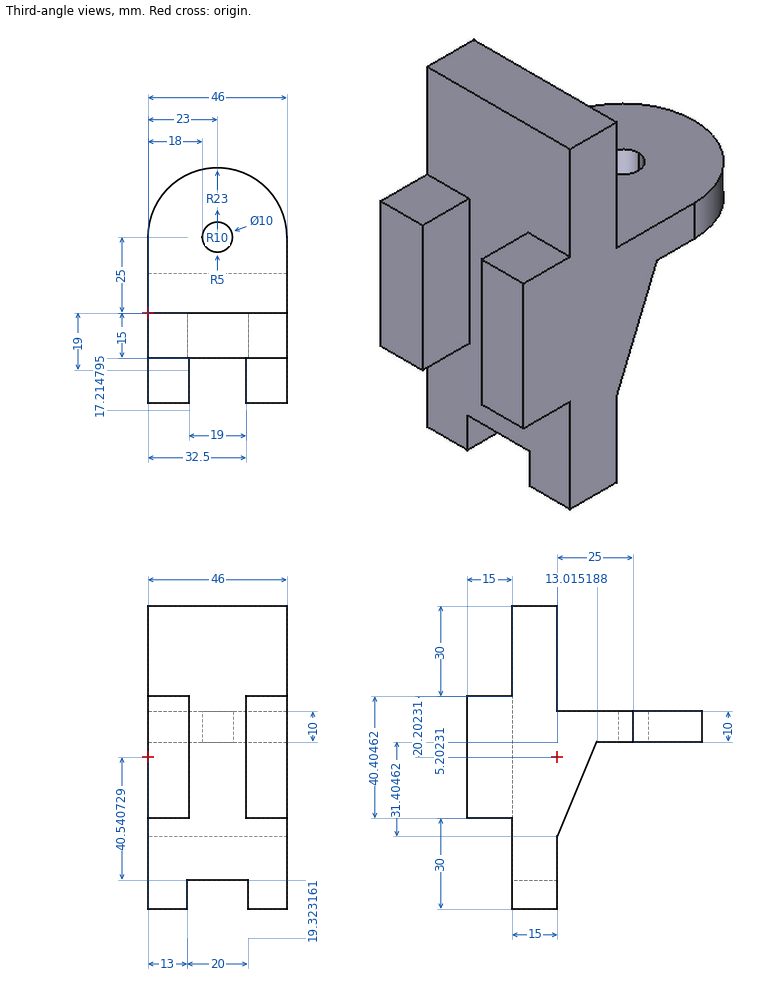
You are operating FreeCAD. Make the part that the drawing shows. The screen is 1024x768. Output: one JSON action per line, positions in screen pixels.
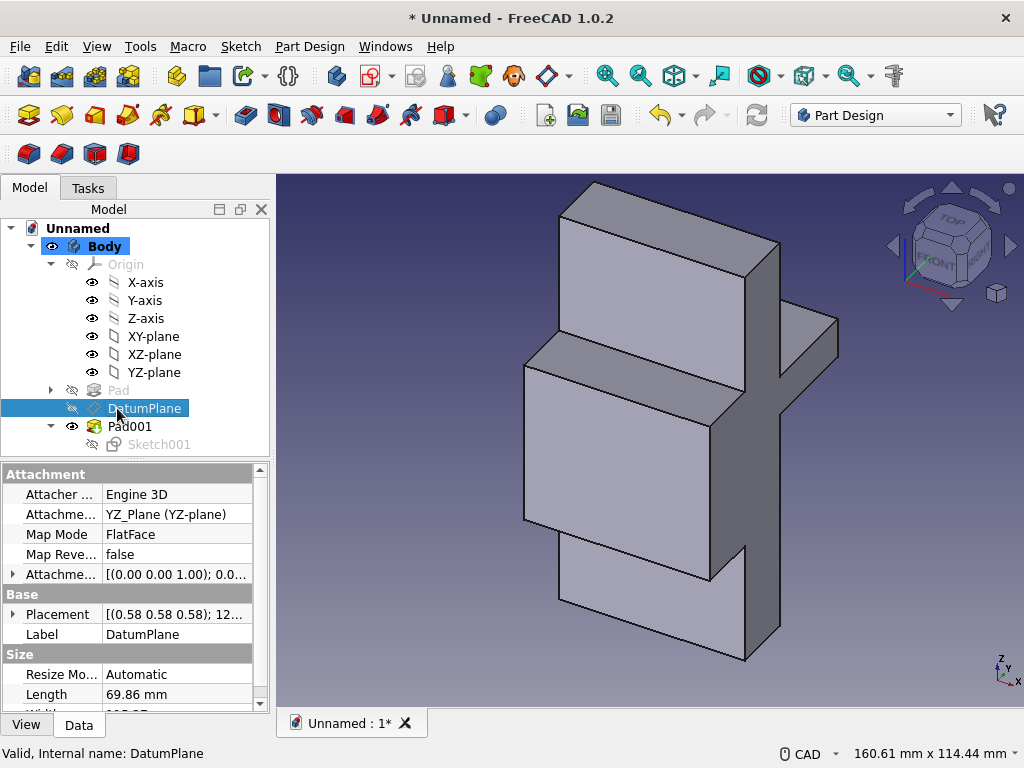
{"action": "left_click", "coordinate": [608, 76]}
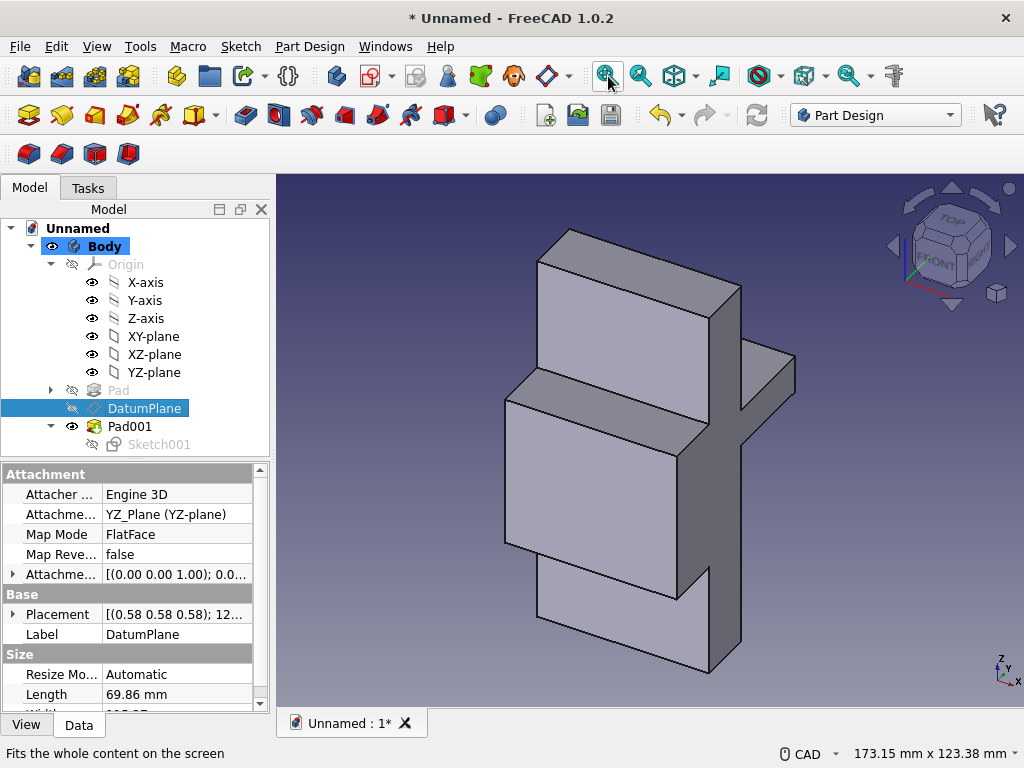
{"action": "left_click", "coordinate": [137, 372]}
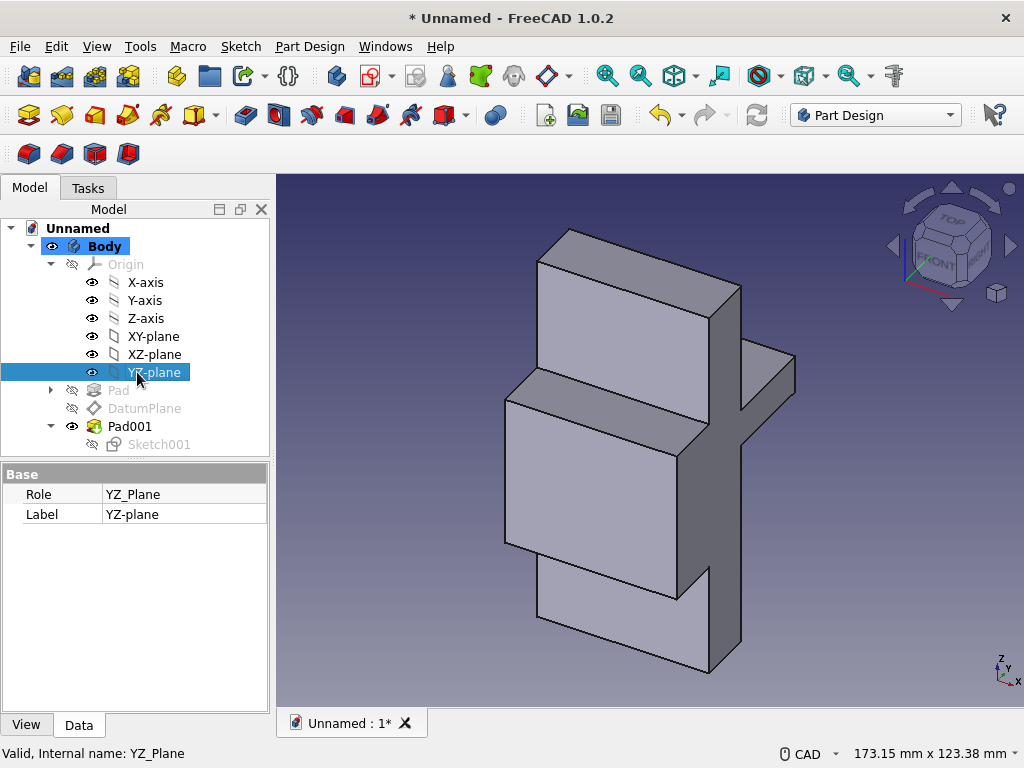
{"action": "left_click", "coordinate": [546, 76]}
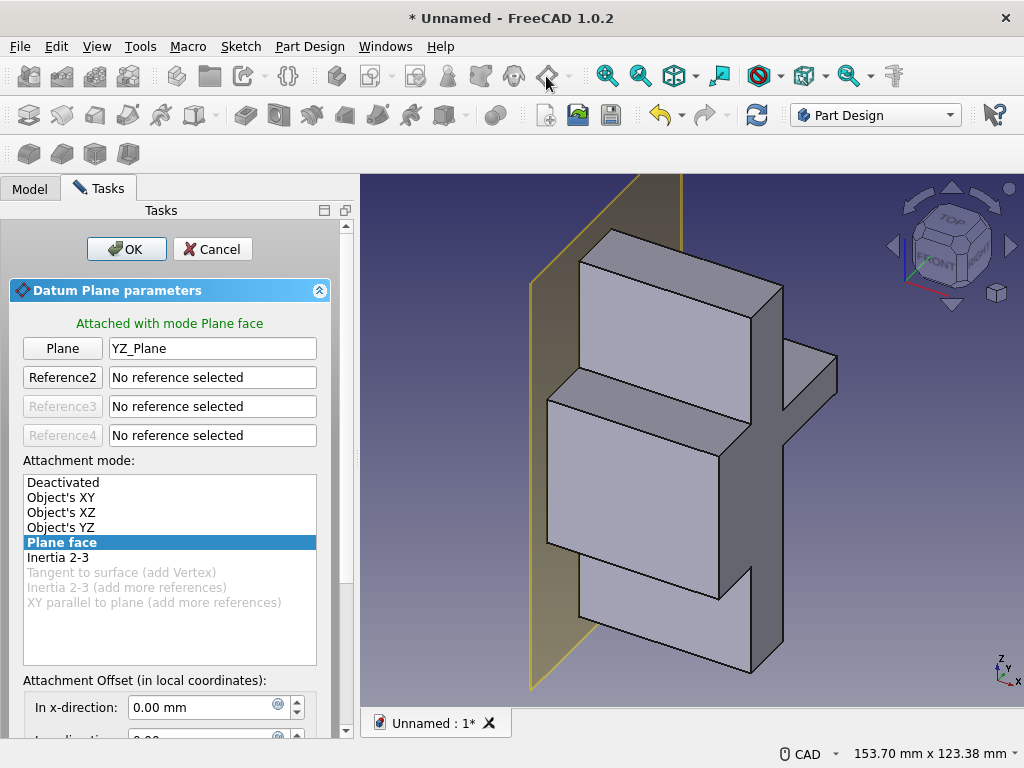
{"action": "scroll", "coordinate": [346, 479], "scroll_direction": "down", "scroll_amount": 2}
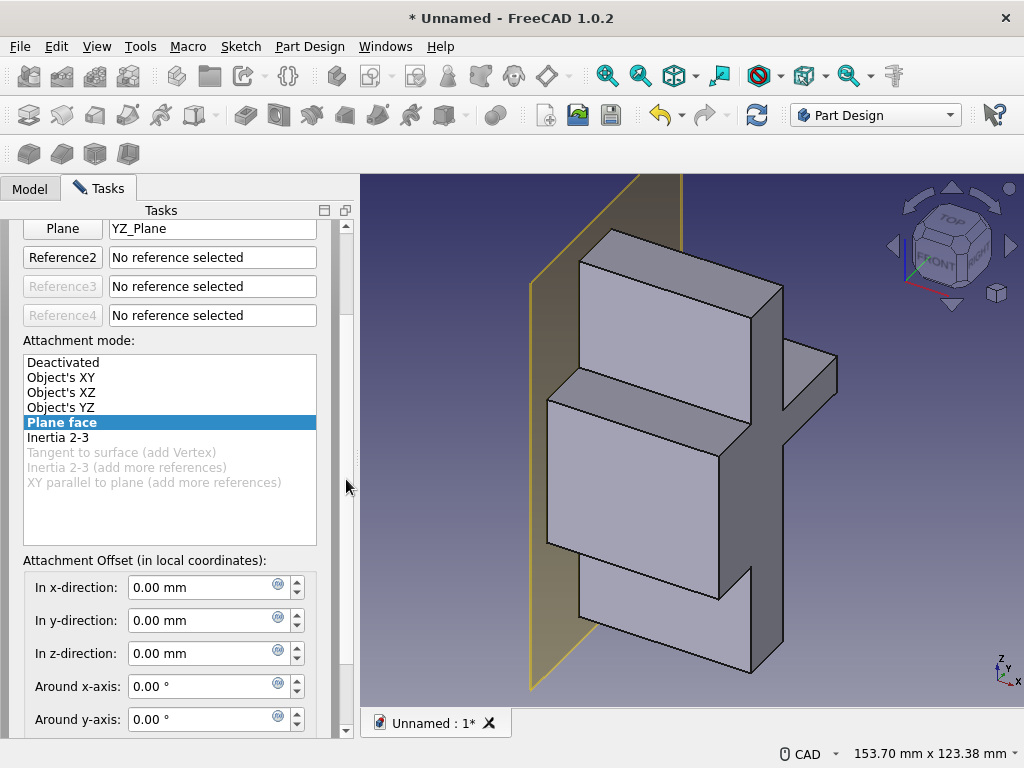
{"action": "triple_click", "coordinate": [210, 654]}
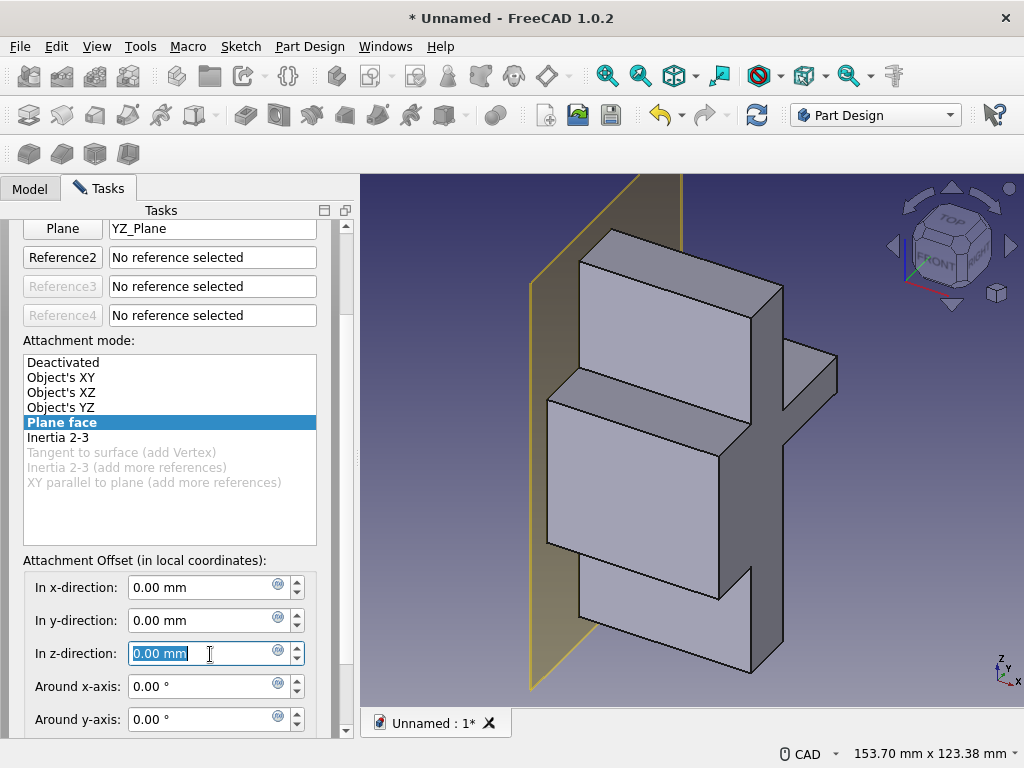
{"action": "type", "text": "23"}
{"action": "key", "text": "Tab"}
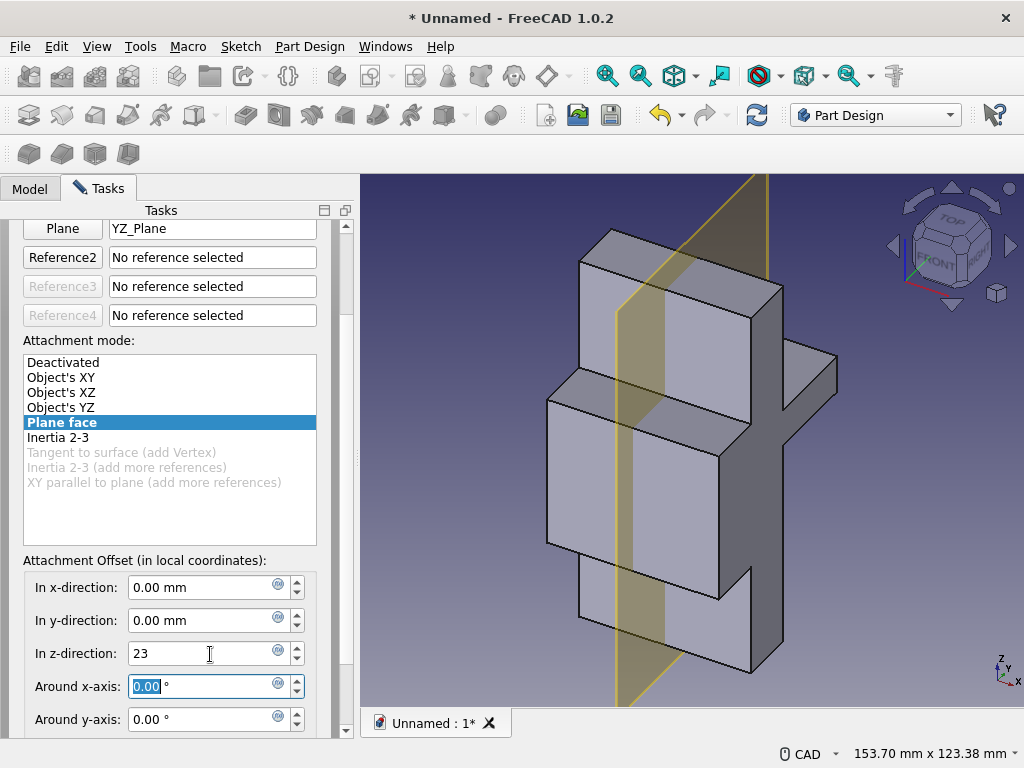
{"action": "scroll", "coordinate": [346, 479], "scroll_direction": "up", "scroll_amount": 3}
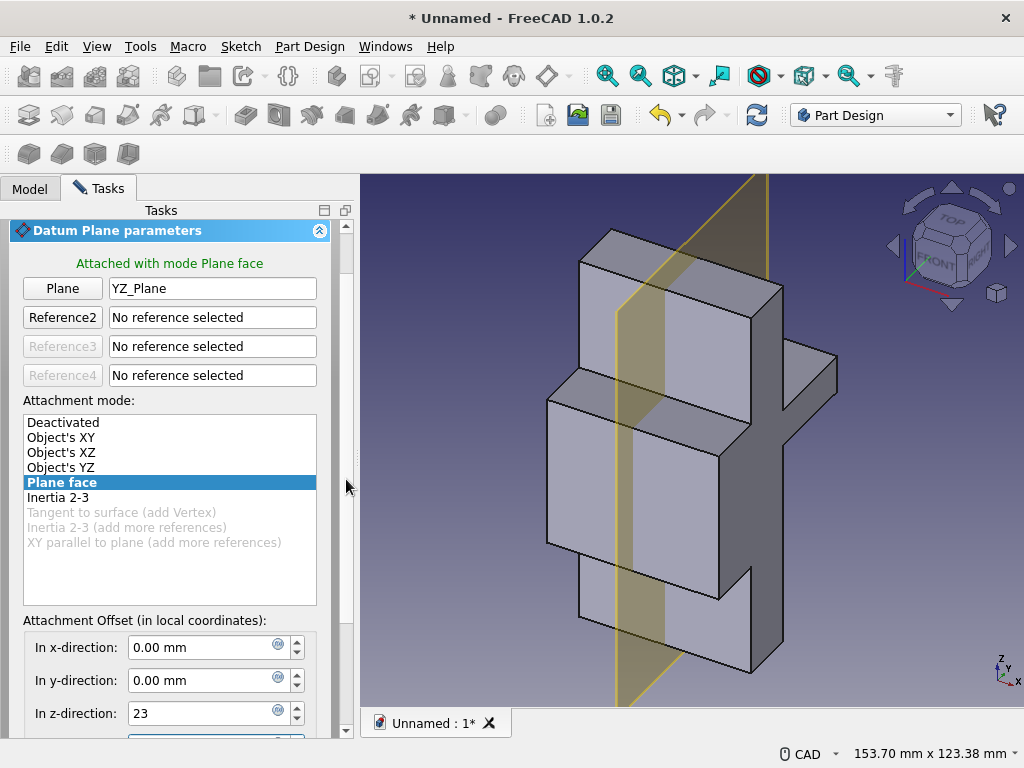
{"action": "left_click", "coordinate": [127, 249]}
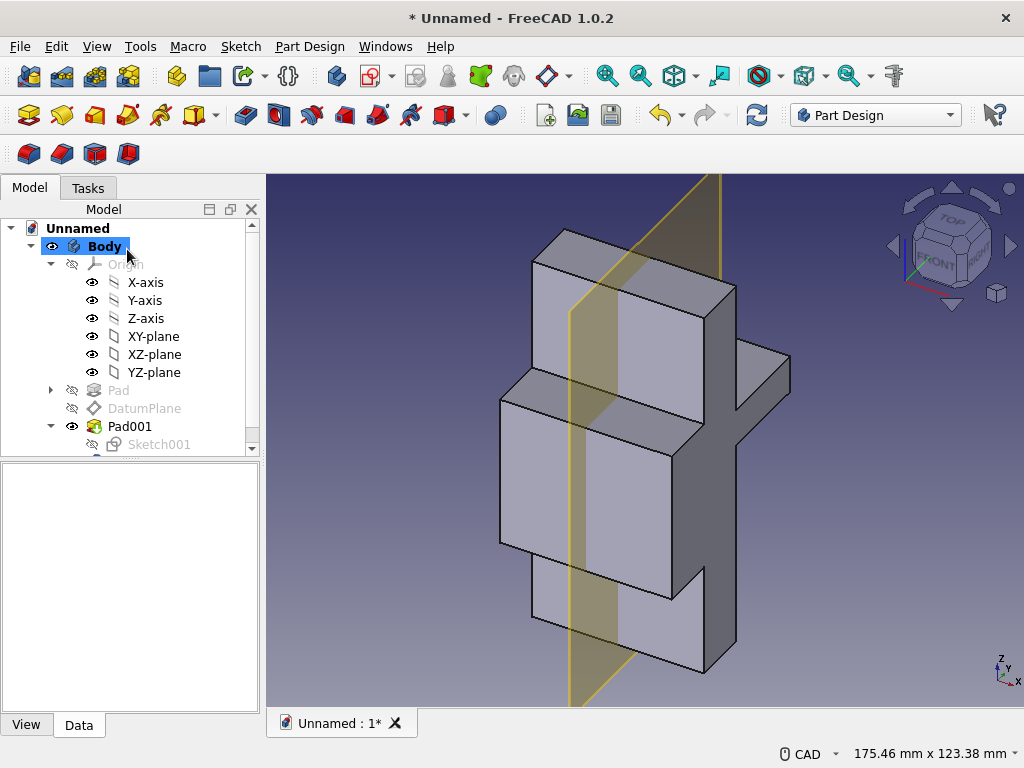
{"action": "scroll", "coordinate": [101, 332], "scroll_direction": "down", "scroll_amount": 3}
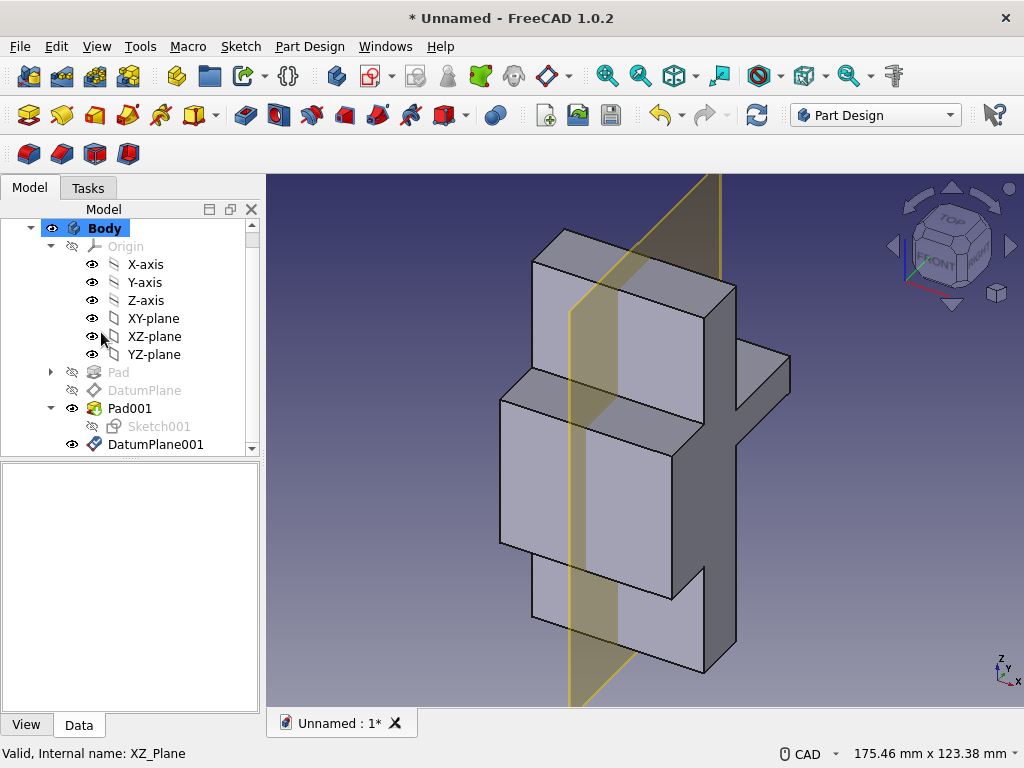
{"action": "left_click", "coordinate": [117, 444]}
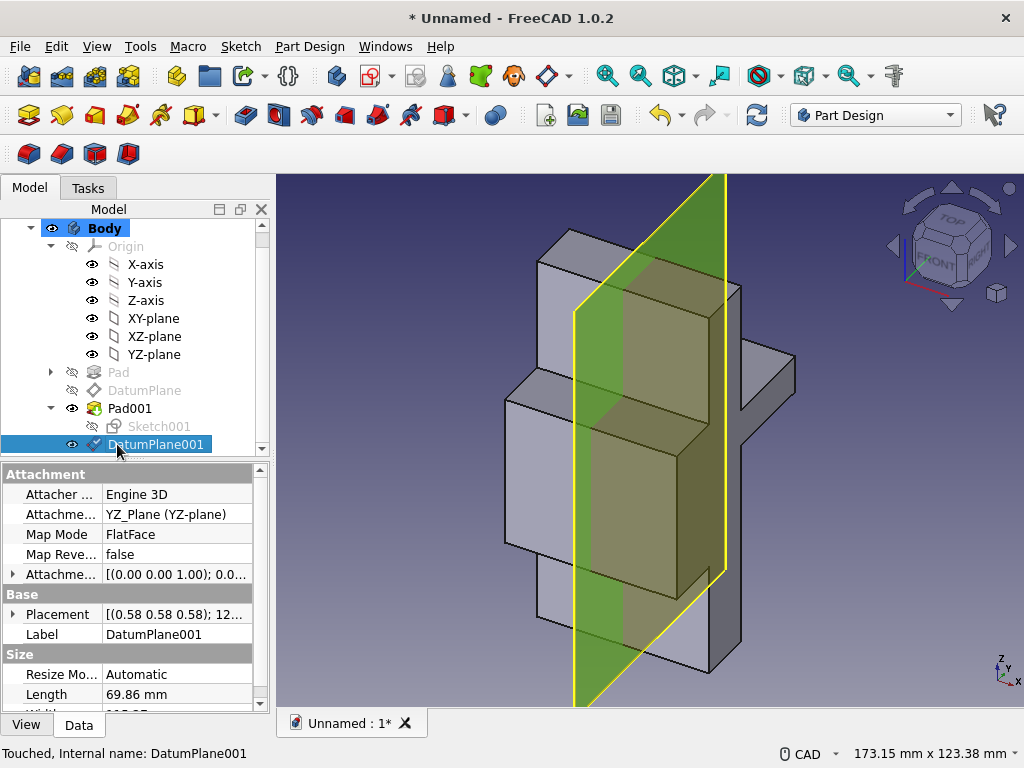
{"action": "left_click", "coordinate": [370, 76]}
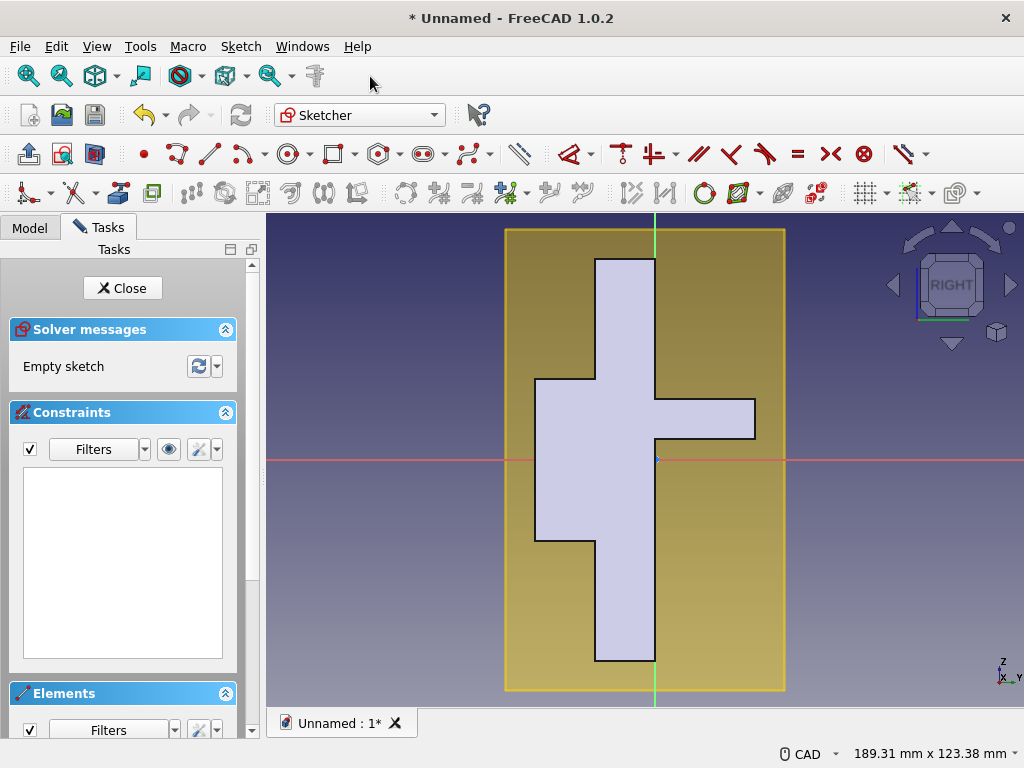
{"action": "key", "text": "q s"}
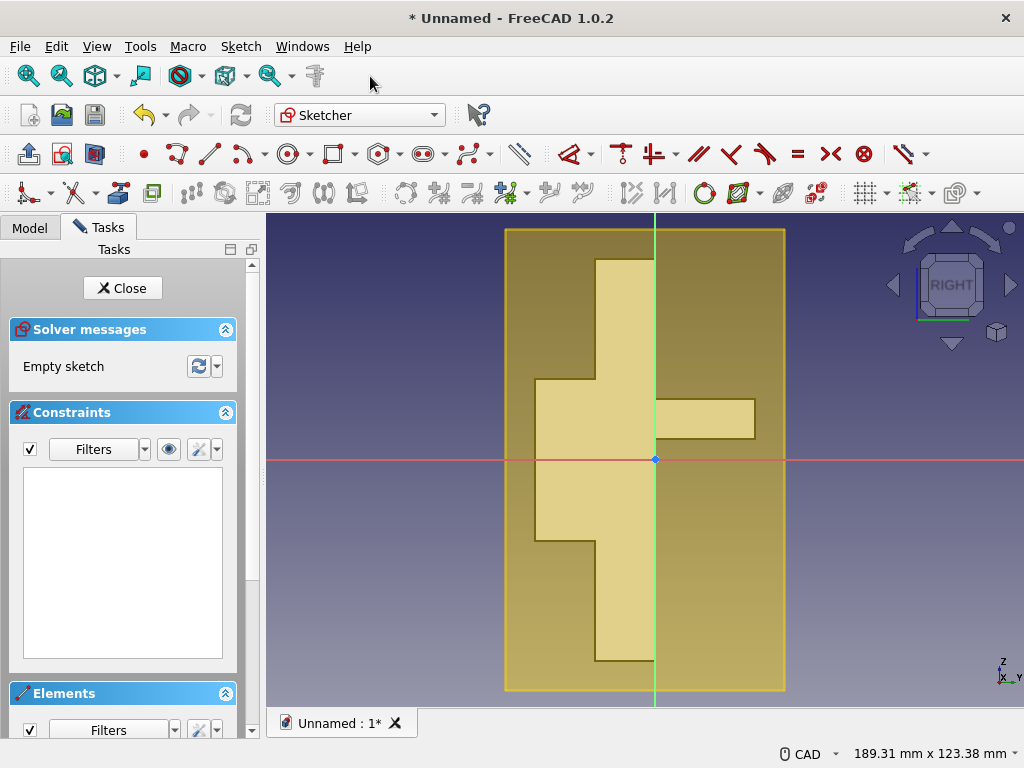
{"action": "scroll", "coordinate": [766, 536], "scroll_direction": "up", "scroll_amount": 4}